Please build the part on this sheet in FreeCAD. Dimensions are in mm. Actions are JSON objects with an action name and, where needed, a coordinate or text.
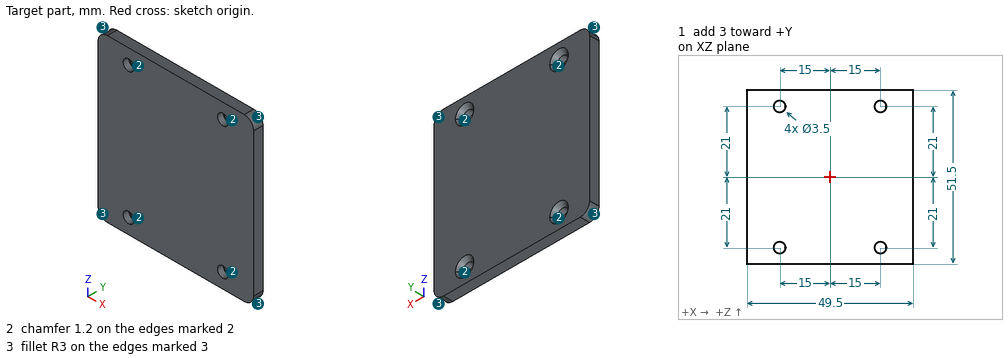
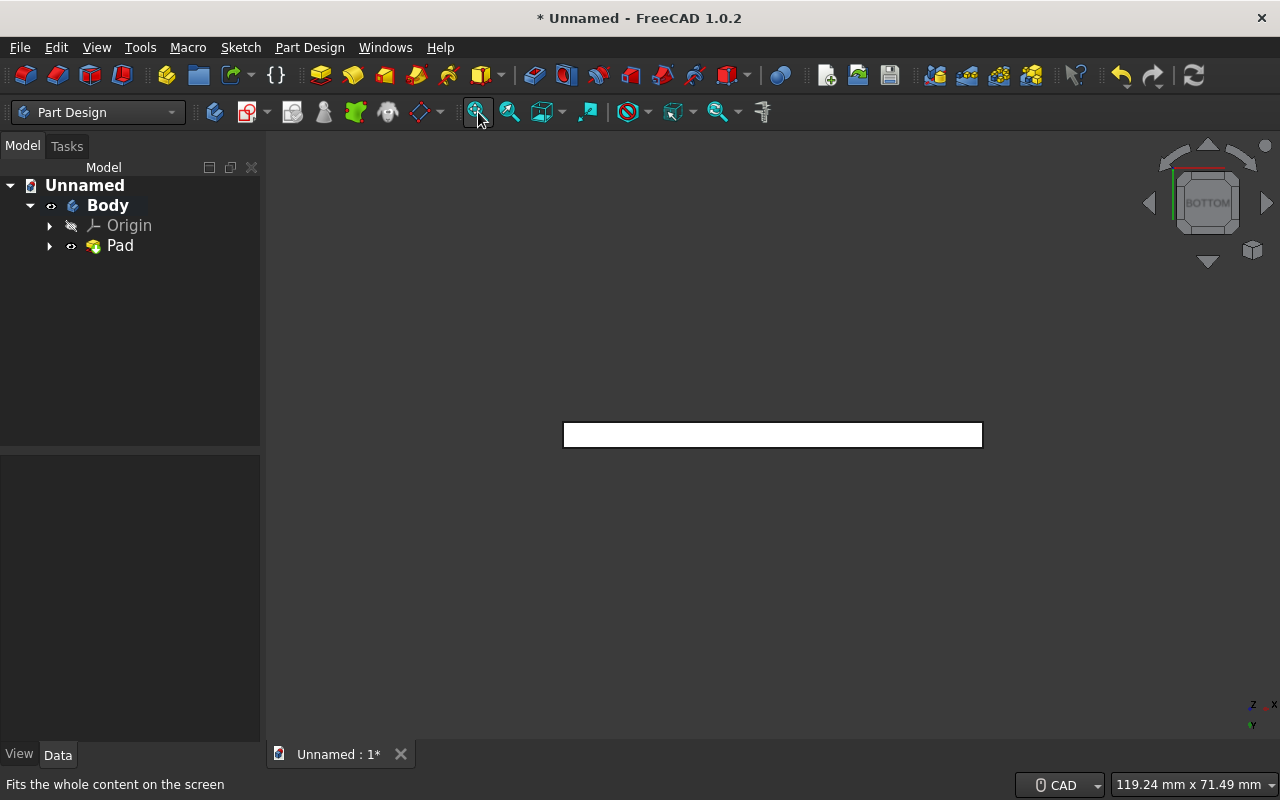
{"action": "key", "text": "4"}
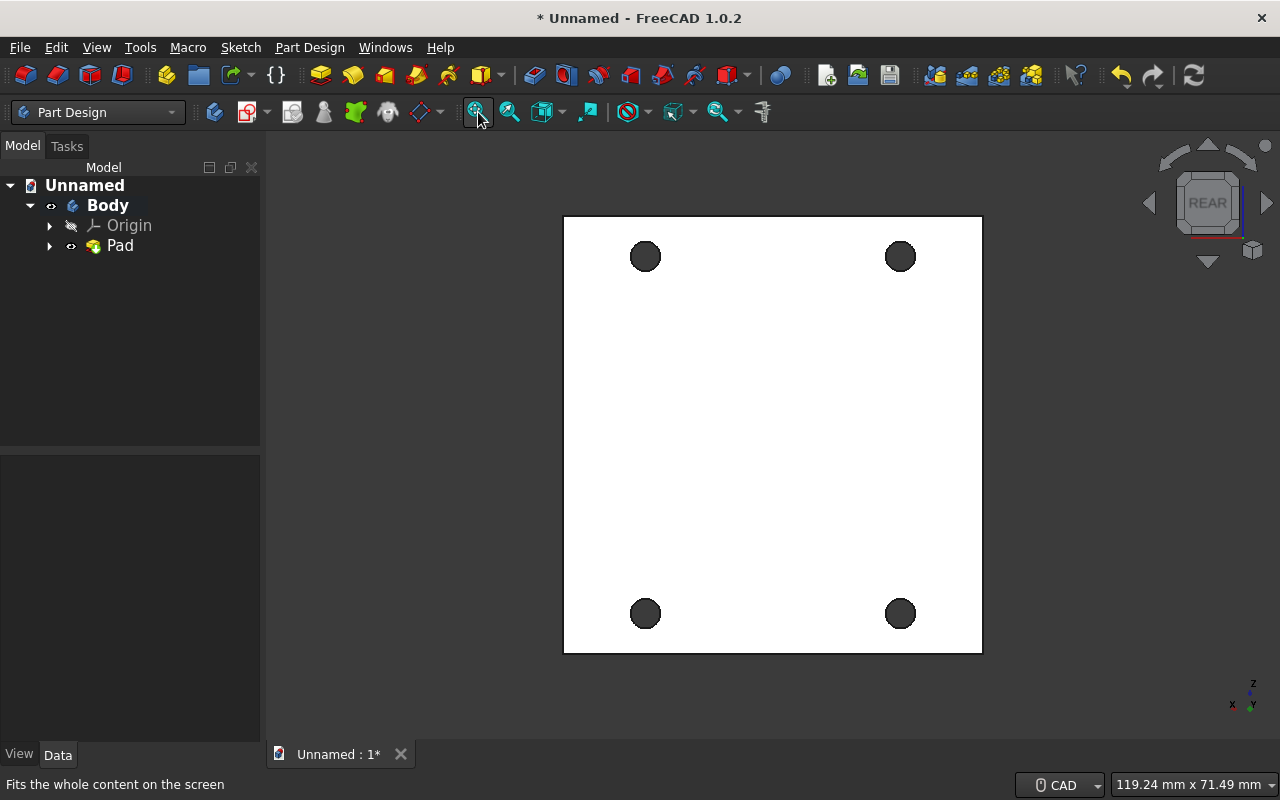
{"action": "left_click", "coordinate": [915, 613]}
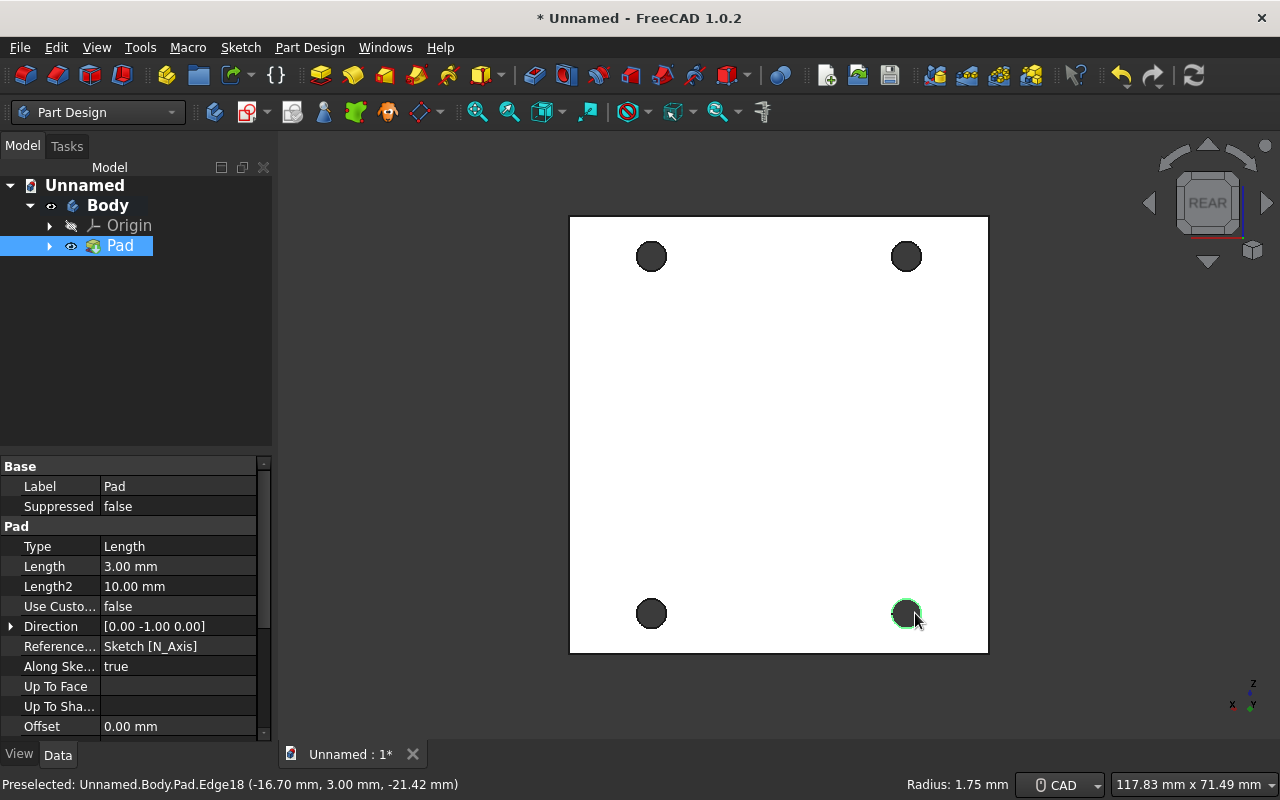
{"action": "left_click", "coordinate": [666, 613], "text": "ctrl"}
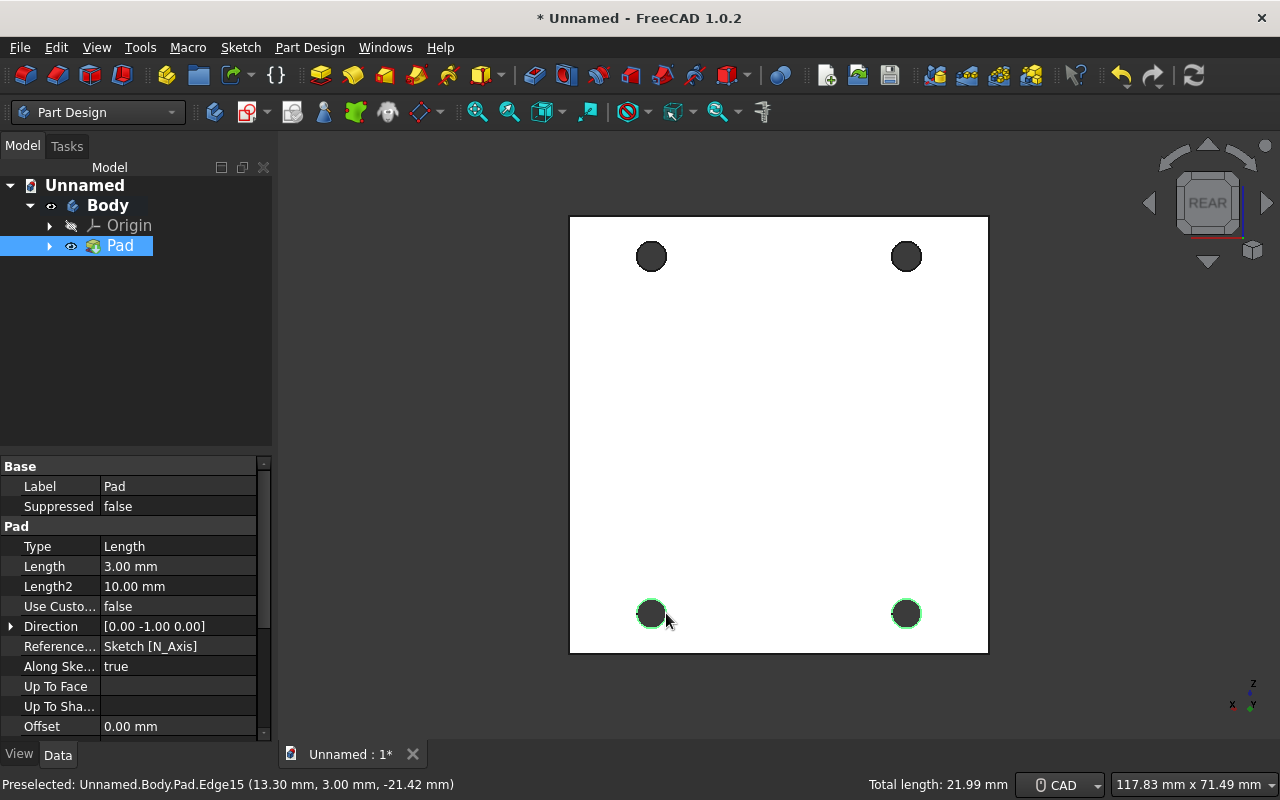
{"action": "left_click", "coordinate": [921, 255], "text": "ctrl"}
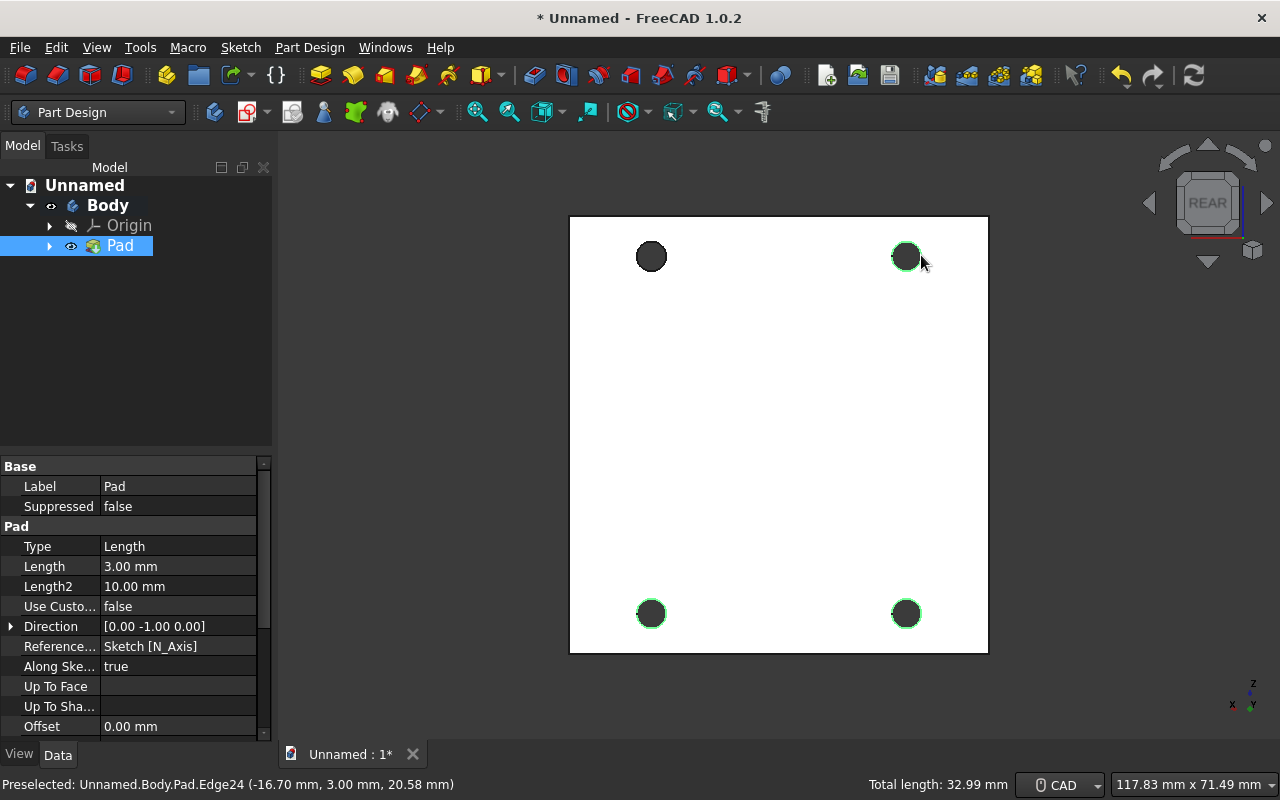
{"action": "left_click", "coordinate": [666, 255], "text": "ctrl"}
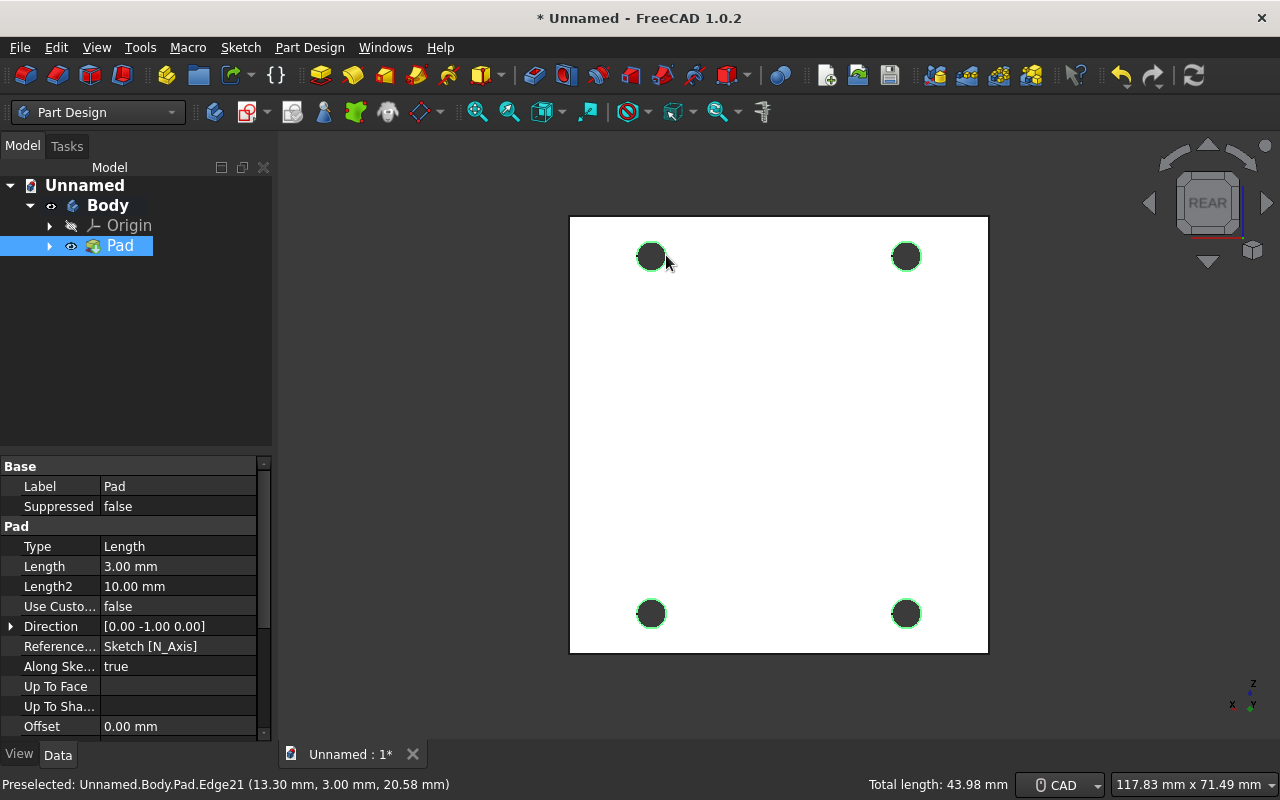
{"action": "left_click", "coordinate": [58, 76]}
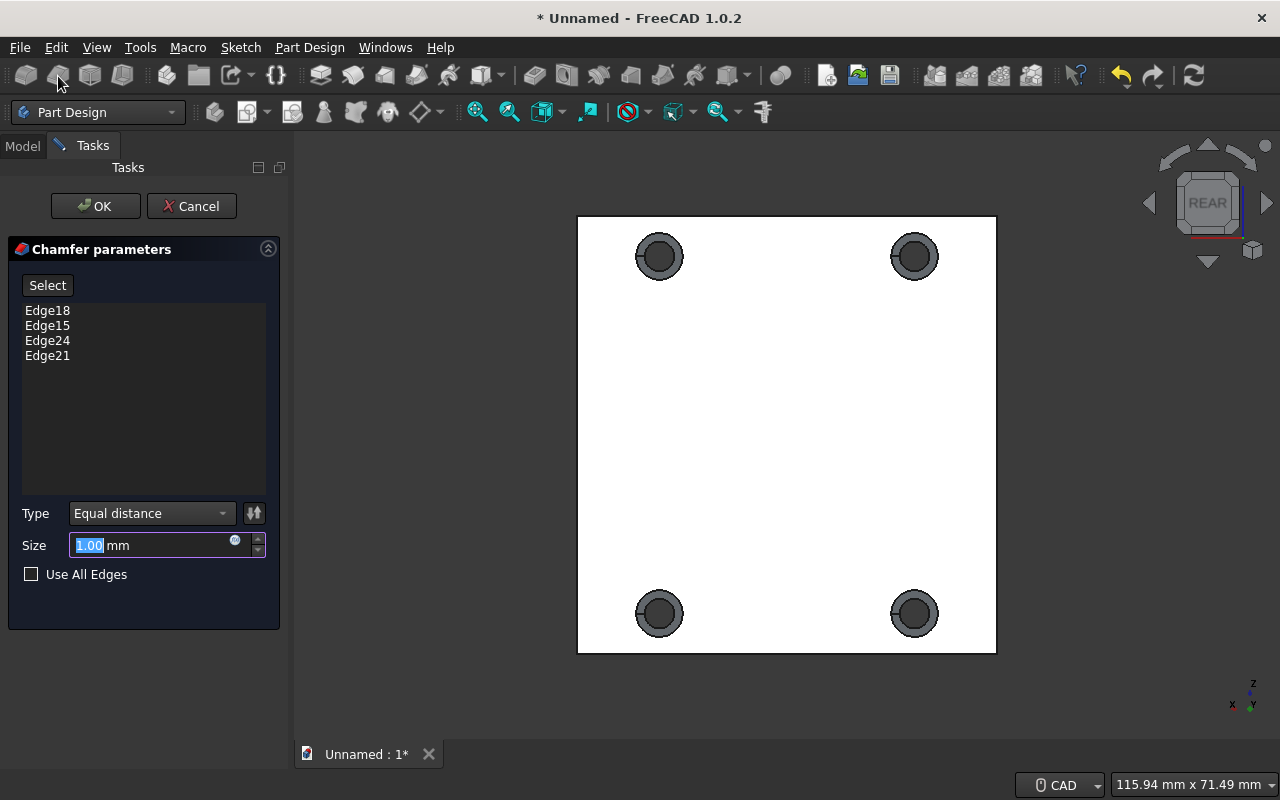
{"action": "type", "text": "1.2"}
{"action": "key", "text": "Tab"}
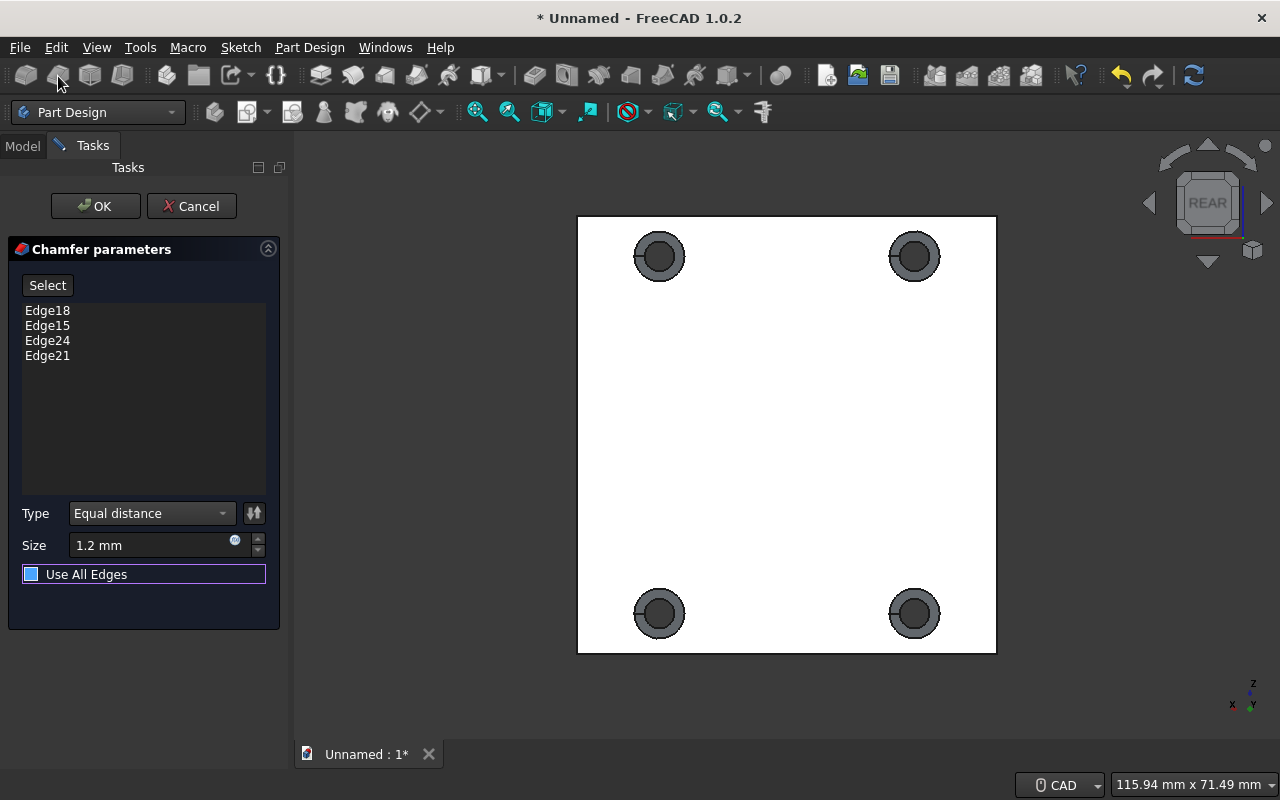
{"action": "left_click", "coordinate": [96, 206]}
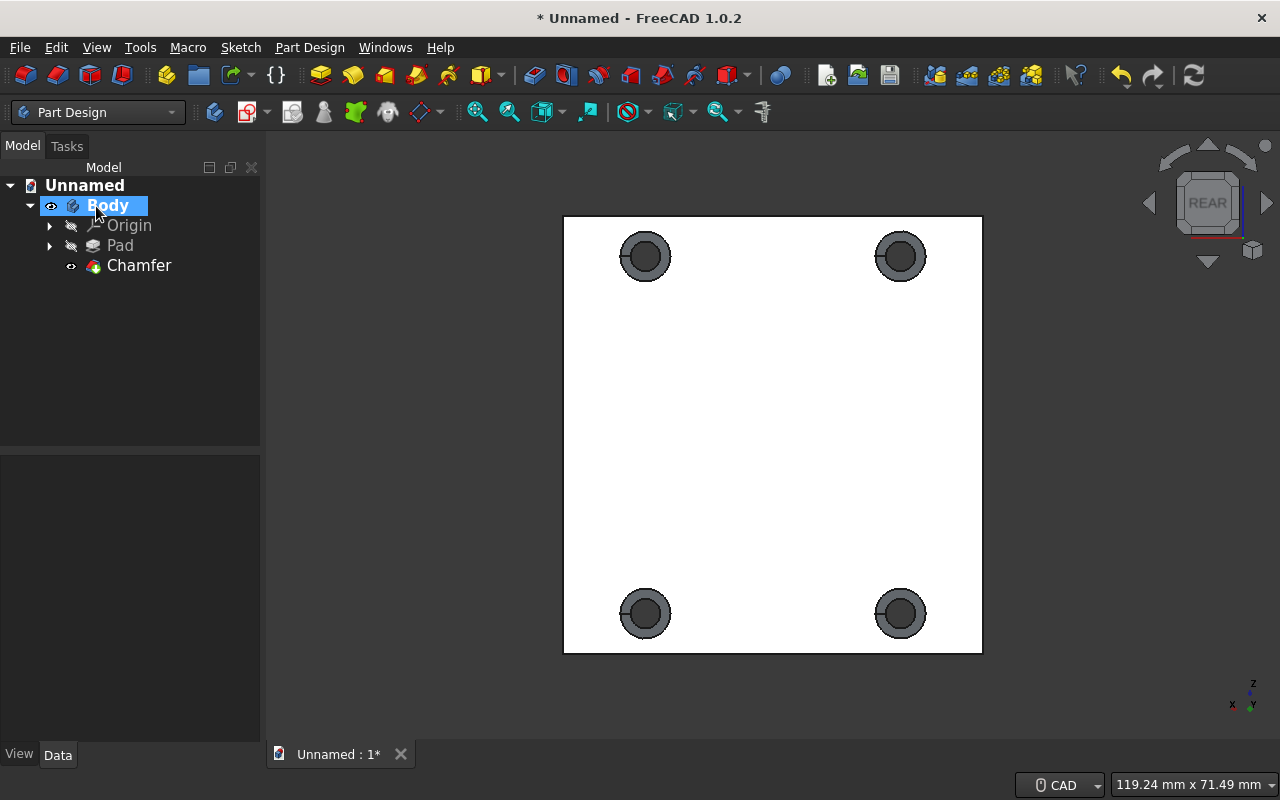
{"action": "key", "text": "0"}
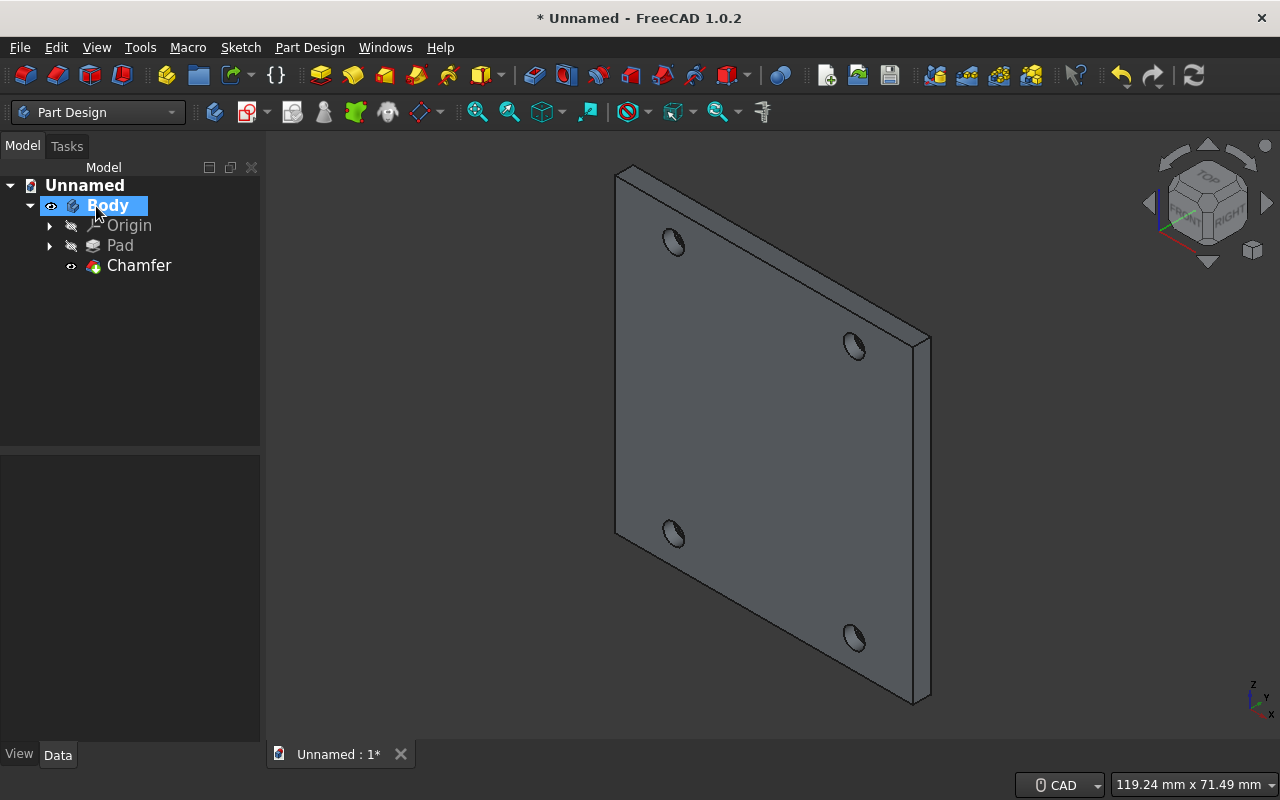
{"action": "left_click", "coordinate": [922, 341]}